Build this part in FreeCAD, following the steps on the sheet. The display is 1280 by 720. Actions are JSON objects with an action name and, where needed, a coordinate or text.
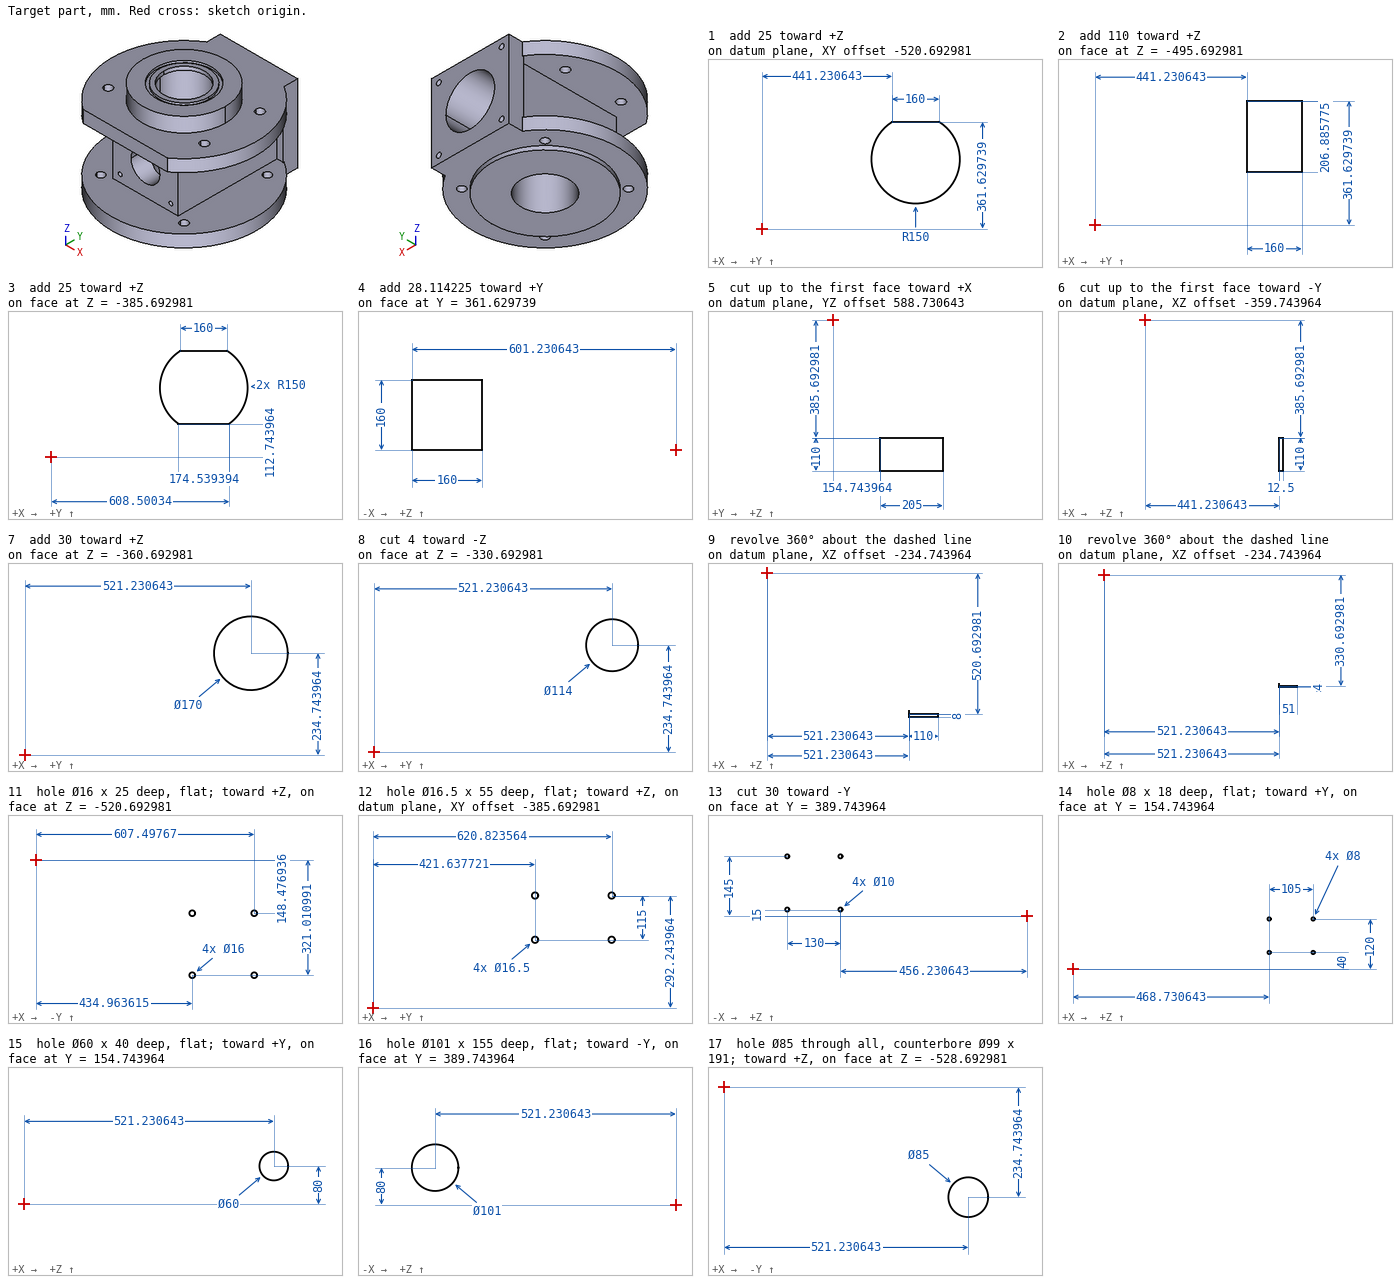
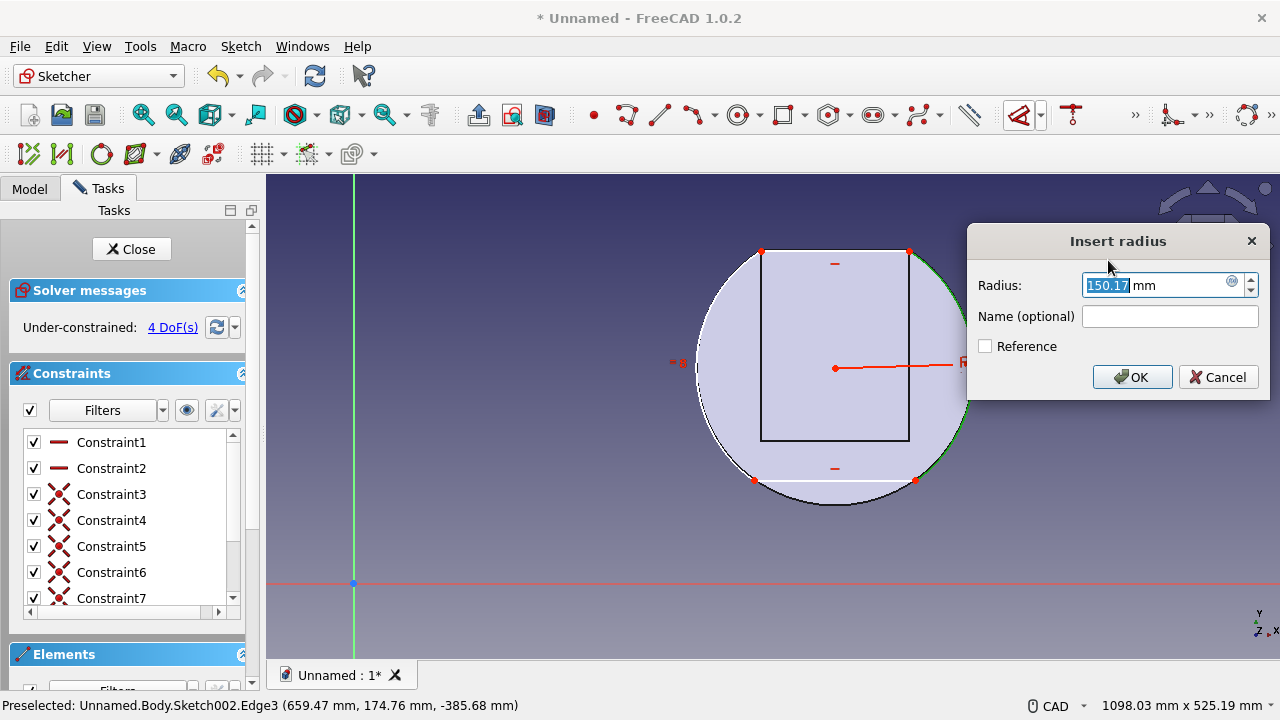
{"action": "type", "text": "150"}
{"action": "key", "text": "Return"}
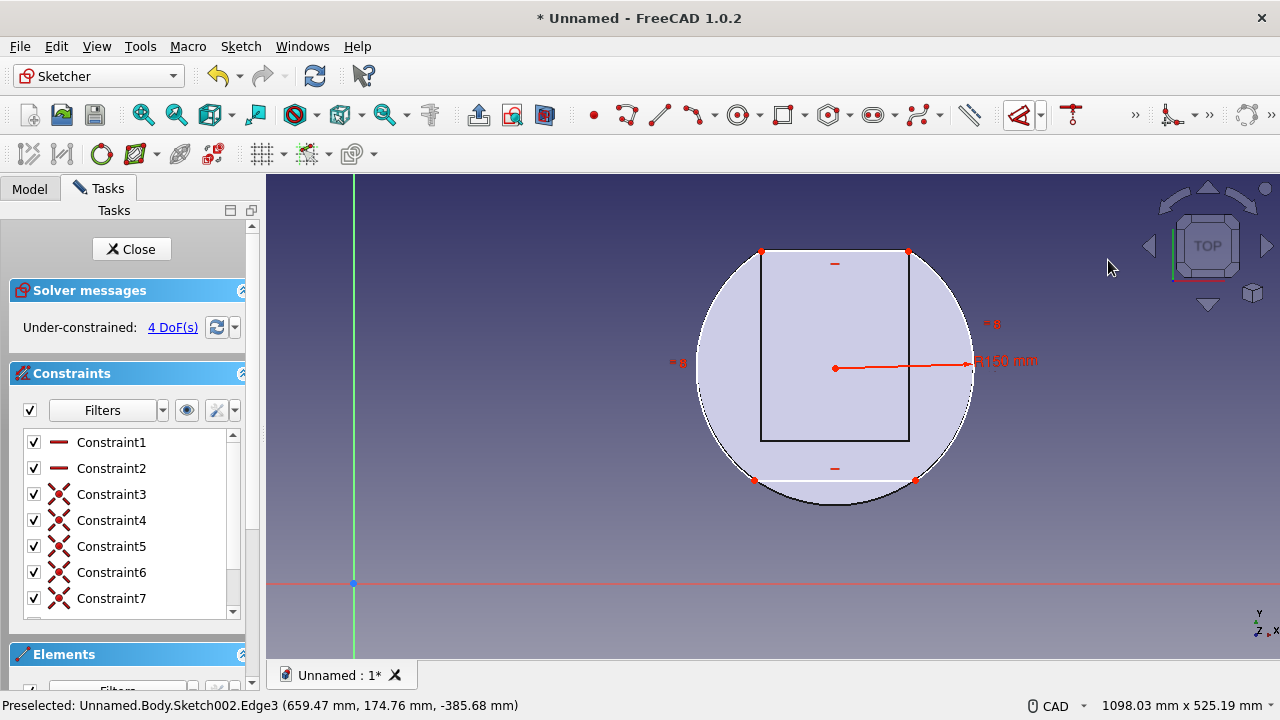
{"action": "left_click", "coordinate": [865, 251]}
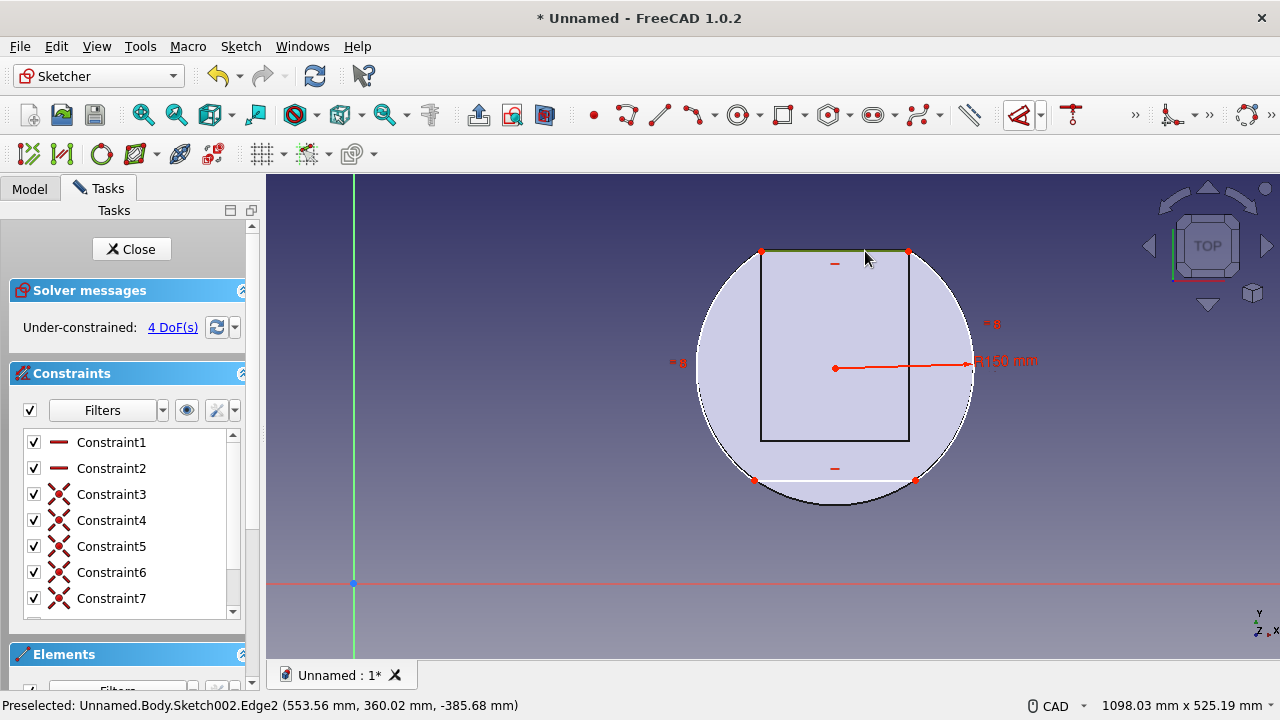
{"action": "key", "text": "l"}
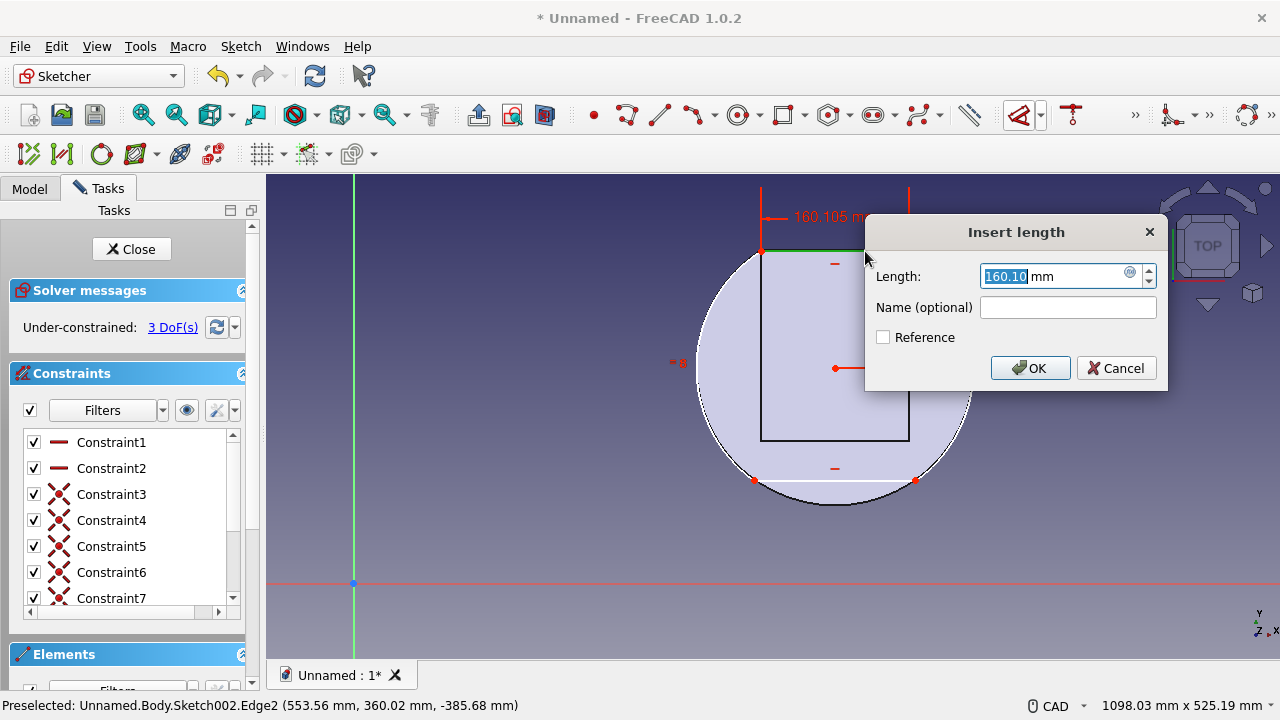
{"action": "type", "text": "160"}
{"action": "key", "text": "Return"}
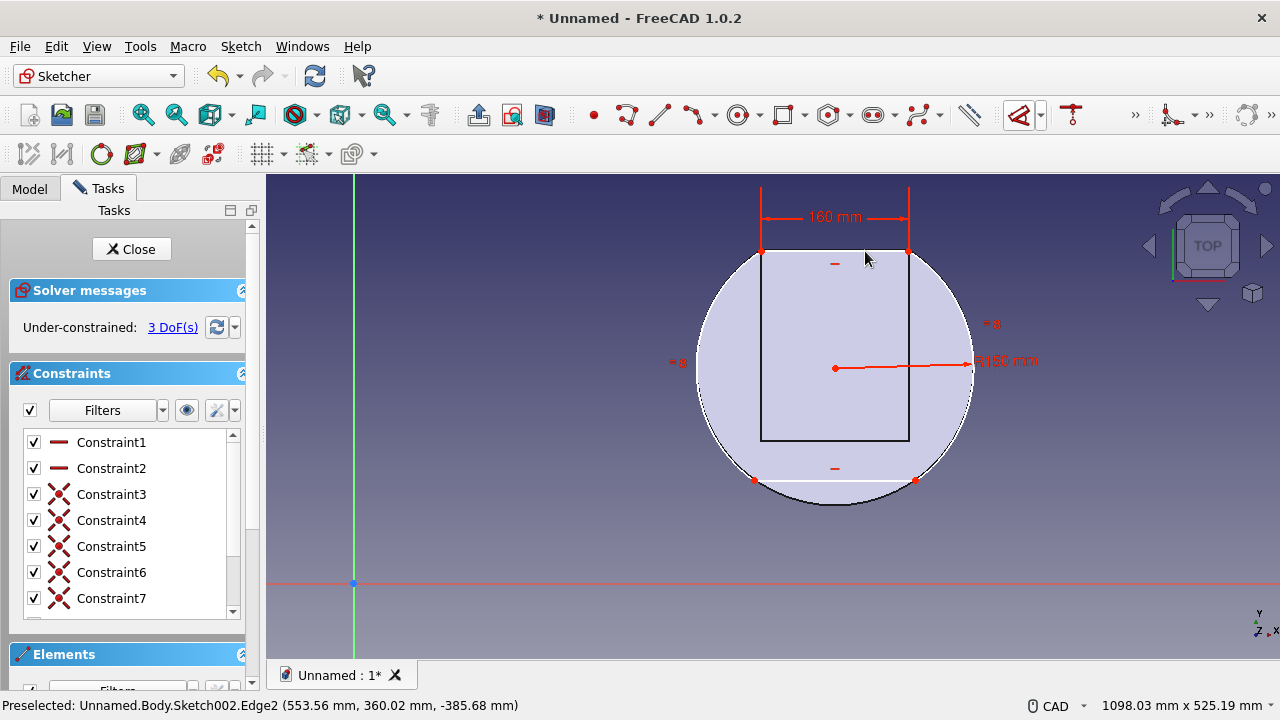
{"action": "left_click", "coordinate": [803, 481]}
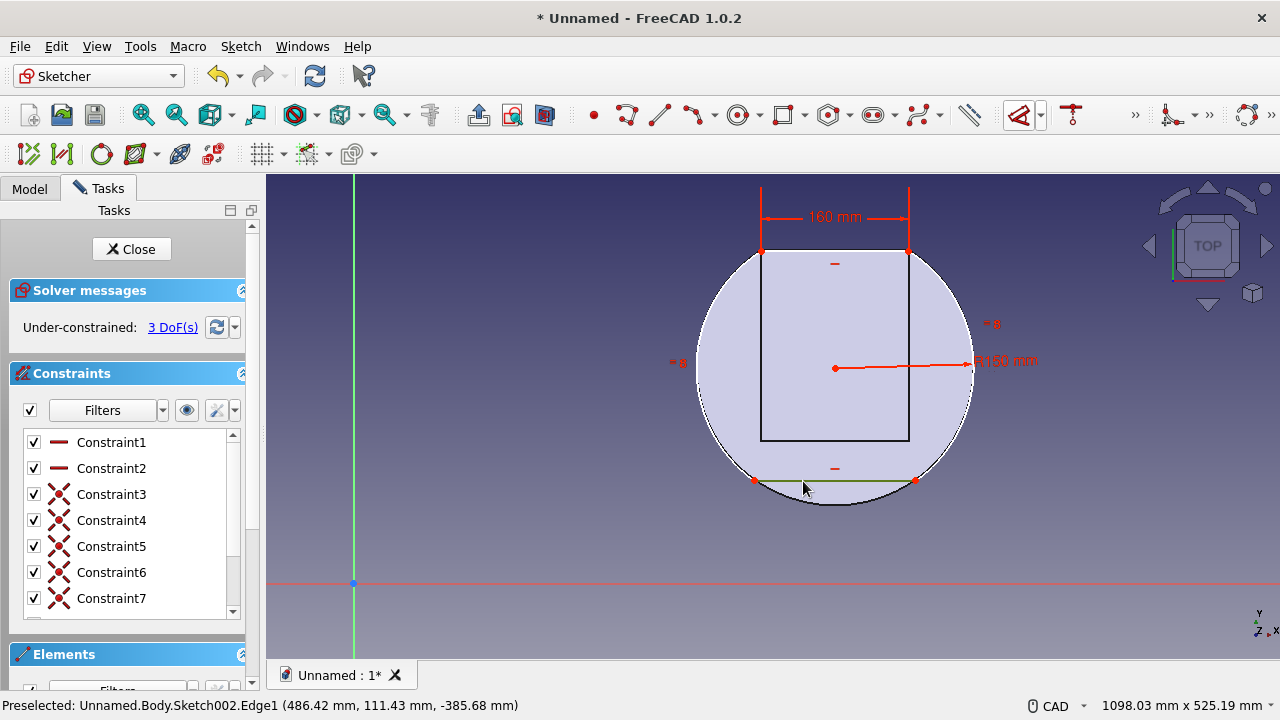
{"action": "key", "text": "l"}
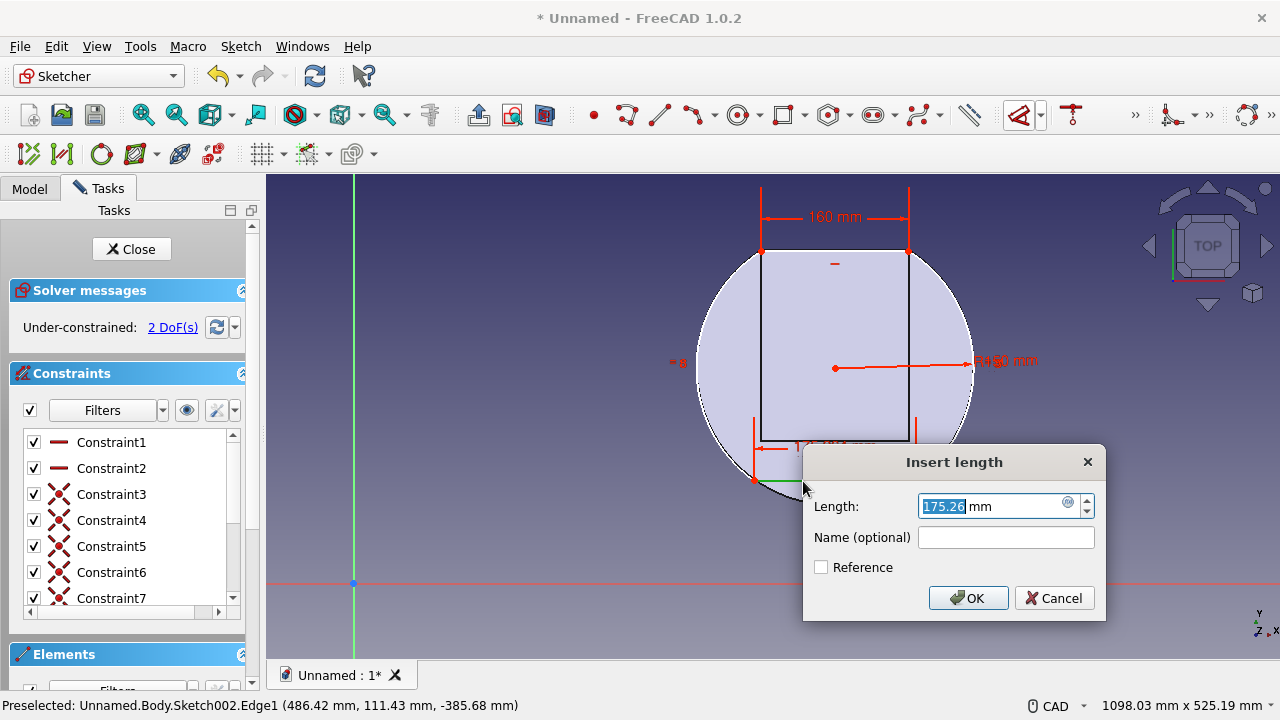
{"action": "type", "text": "174.539394"}
{"action": "key", "text": "Return"}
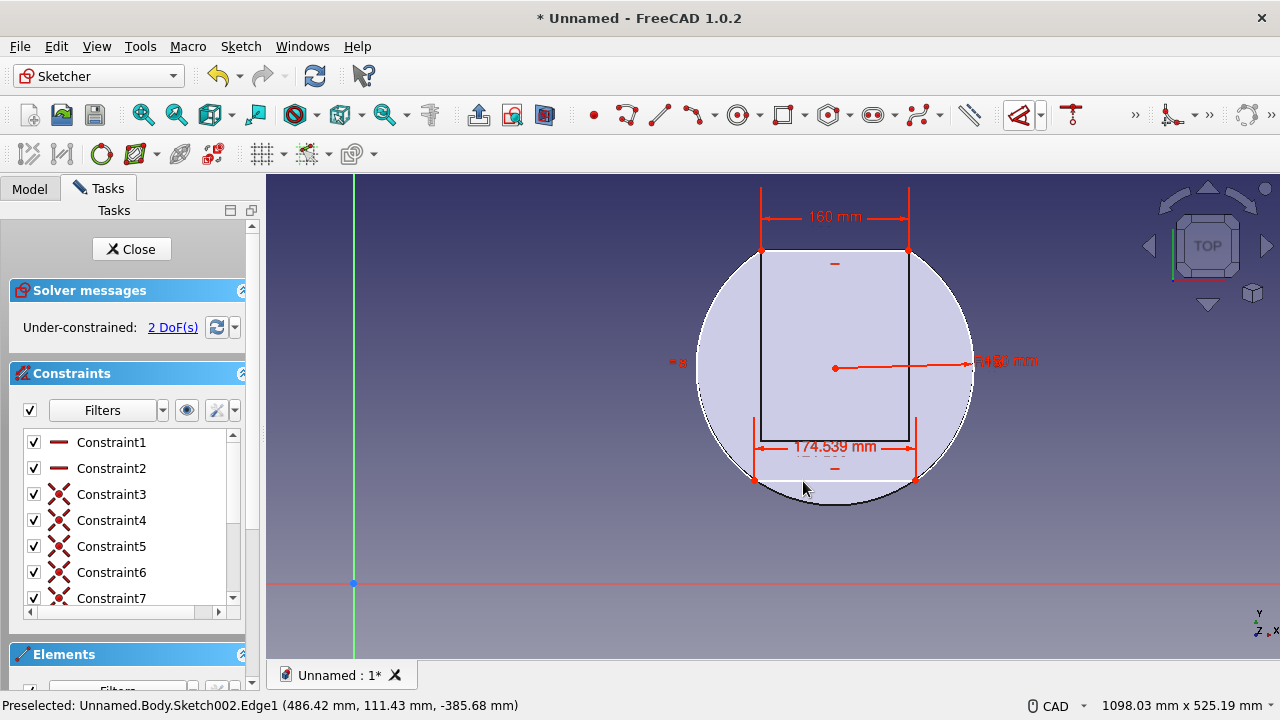
{"action": "left_click", "coordinate": [916, 481]}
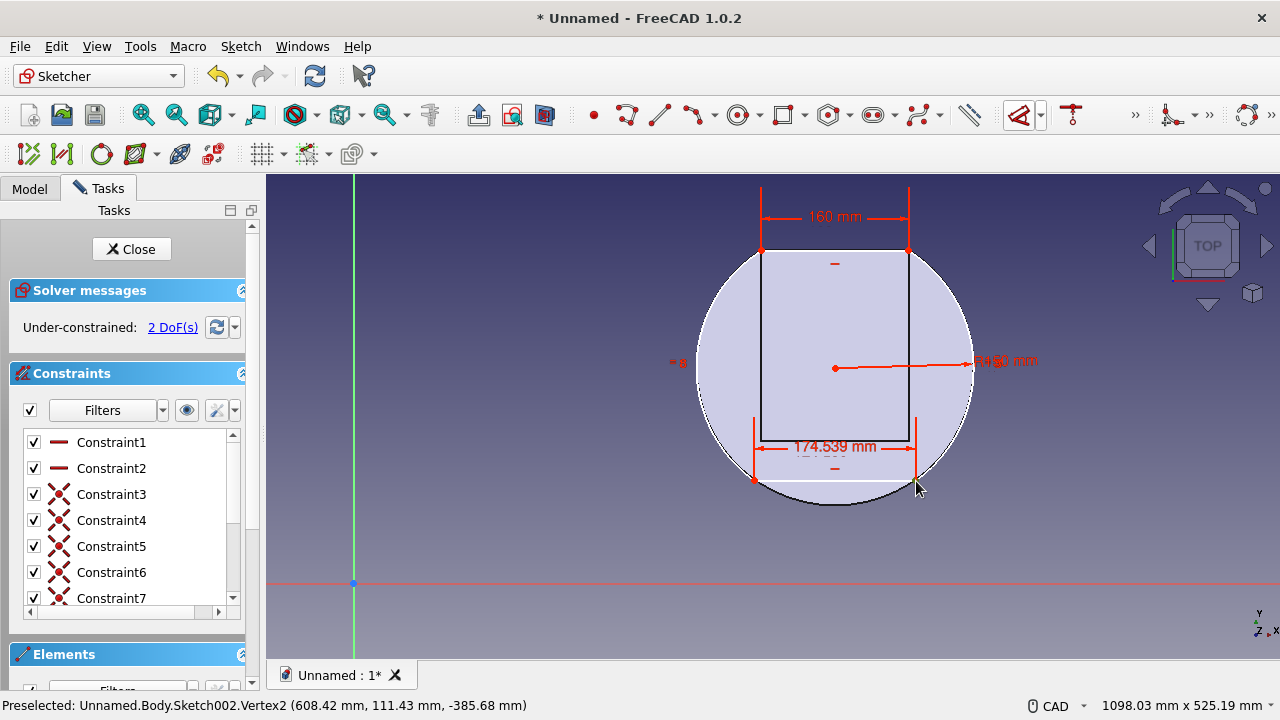
{"action": "key", "text": "l"}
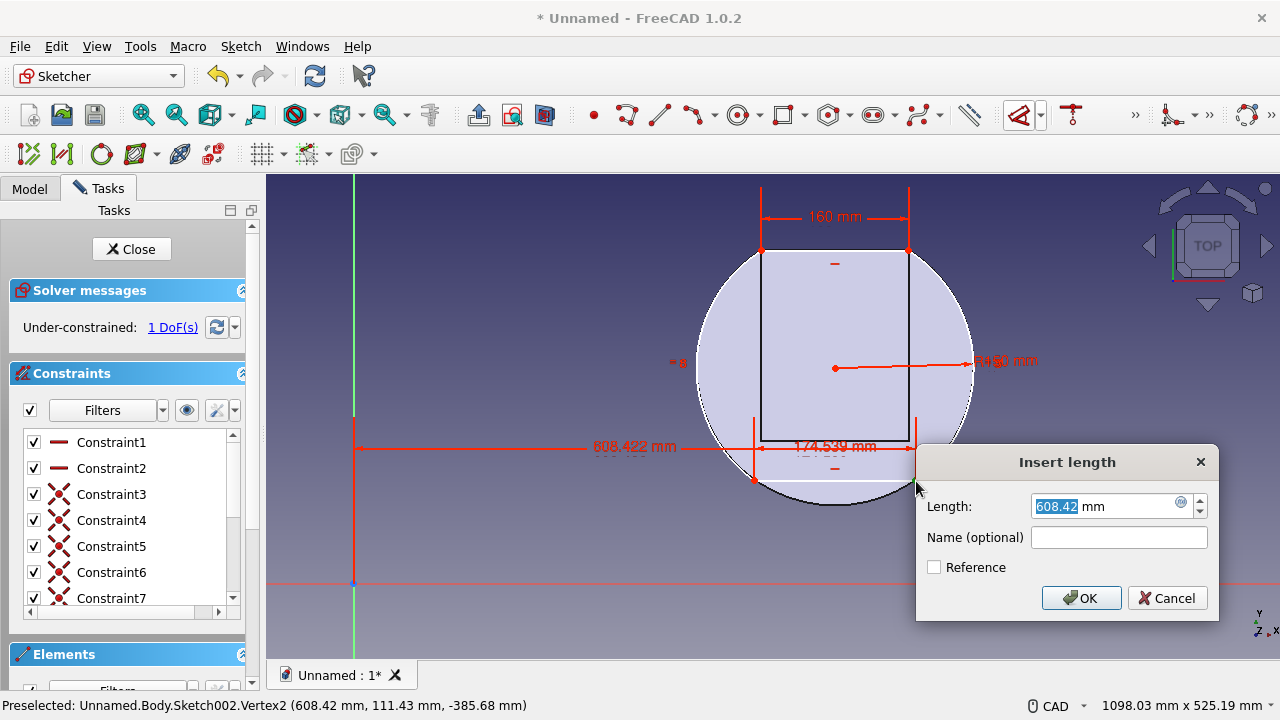
{"action": "type", "text": "608.50034"}
{"action": "key", "text": "Return"}